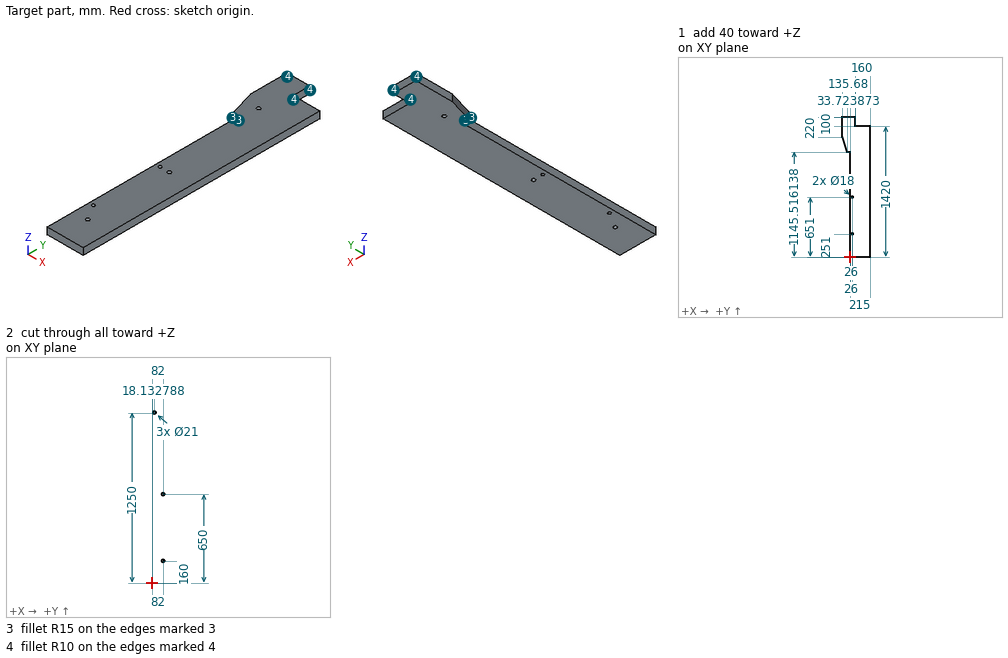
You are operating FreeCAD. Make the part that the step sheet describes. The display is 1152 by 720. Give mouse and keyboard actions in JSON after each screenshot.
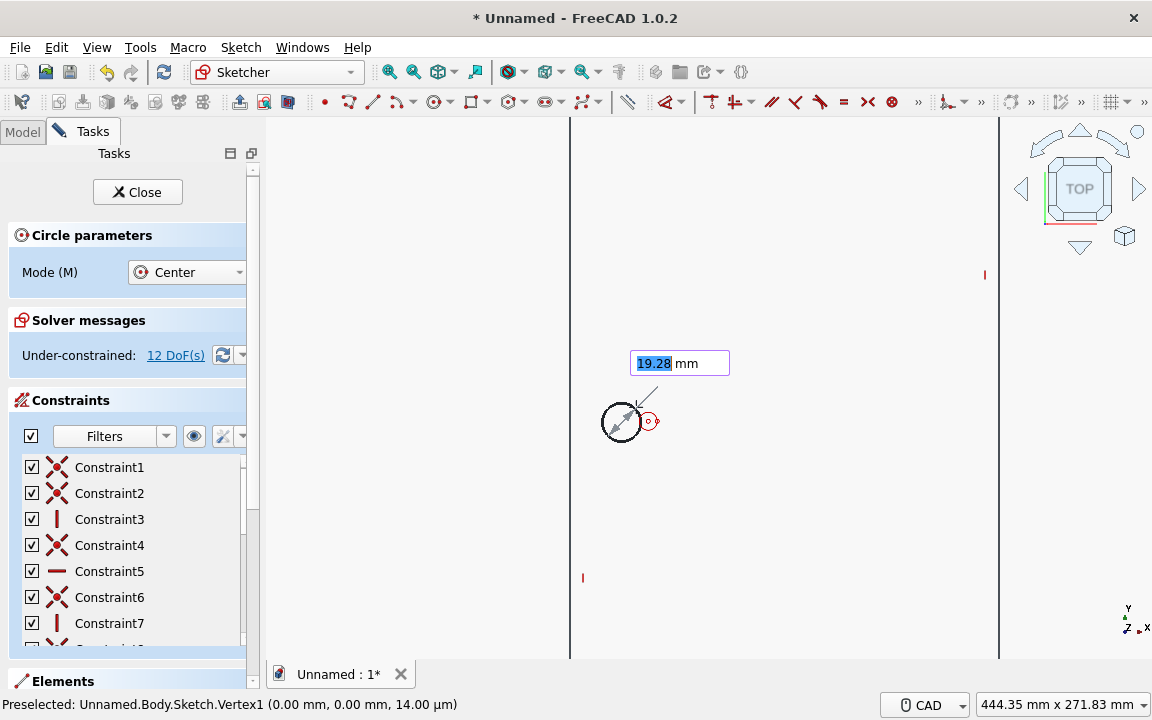
{"action": "left_click", "coordinate": [635, 406]}
{"action": "key", "text": "Escape"}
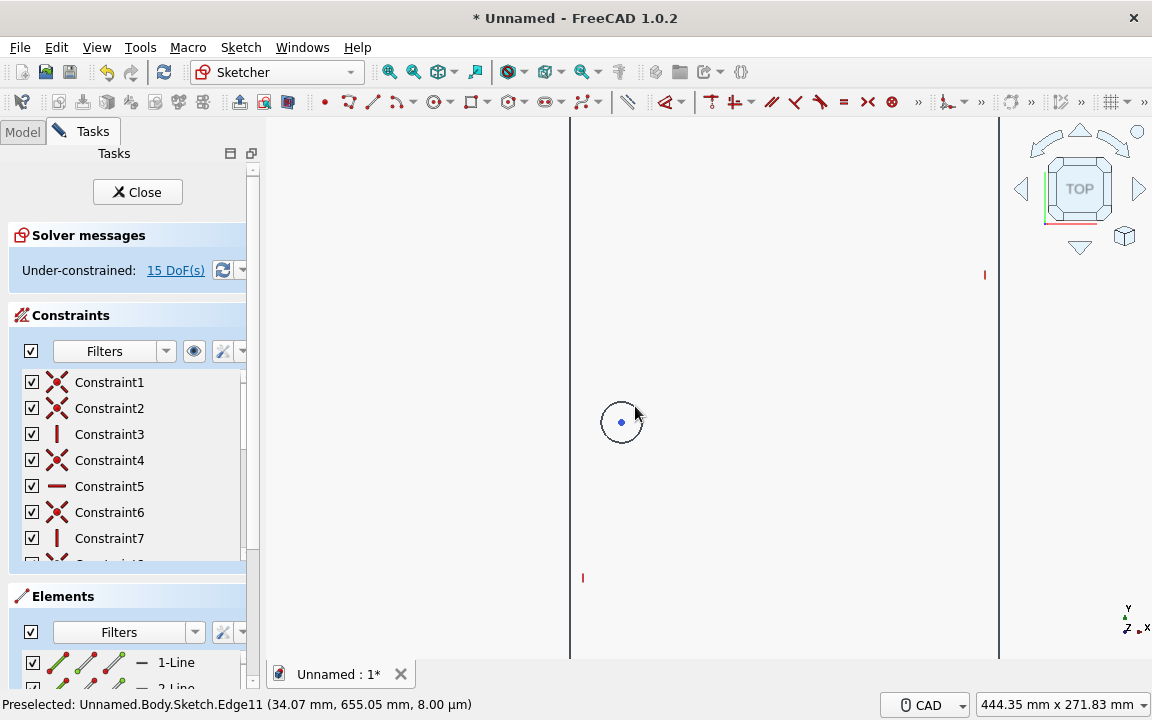
{"action": "scroll", "coordinate": [633, 411], "scroll_direction": "down", "scroll_amount": 11}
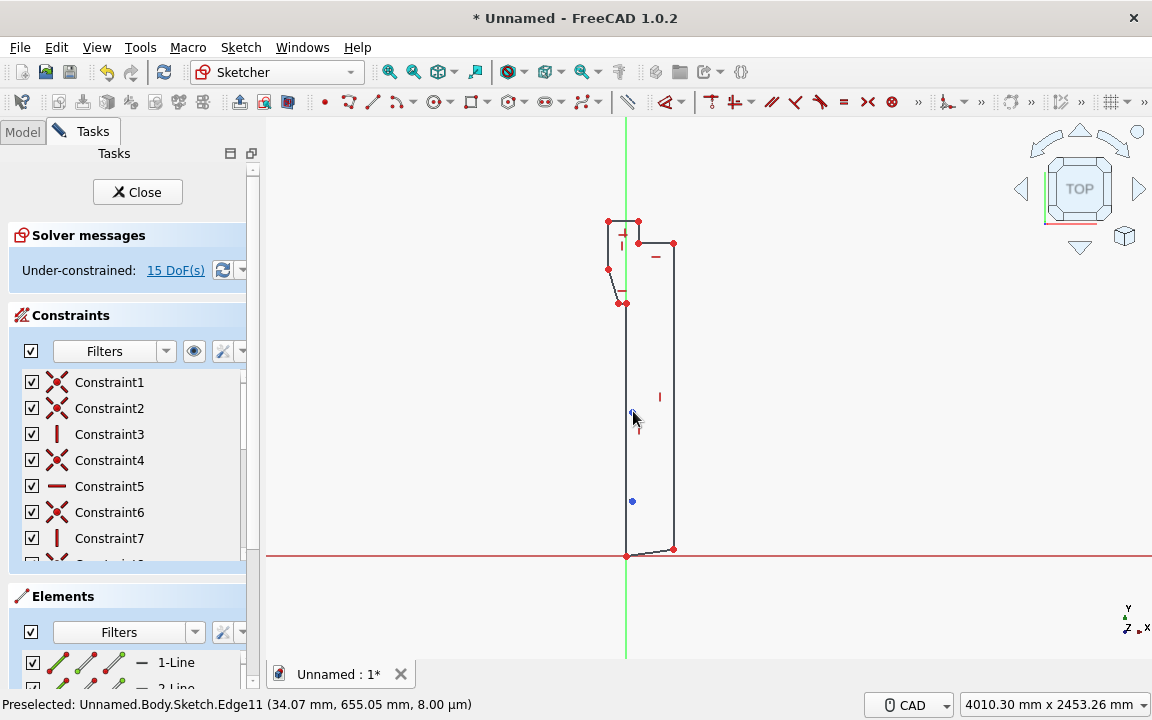
{"action": "scroll", "coordinate": [641, 554], "scroll_direction": "up", "scroll_amount": 10}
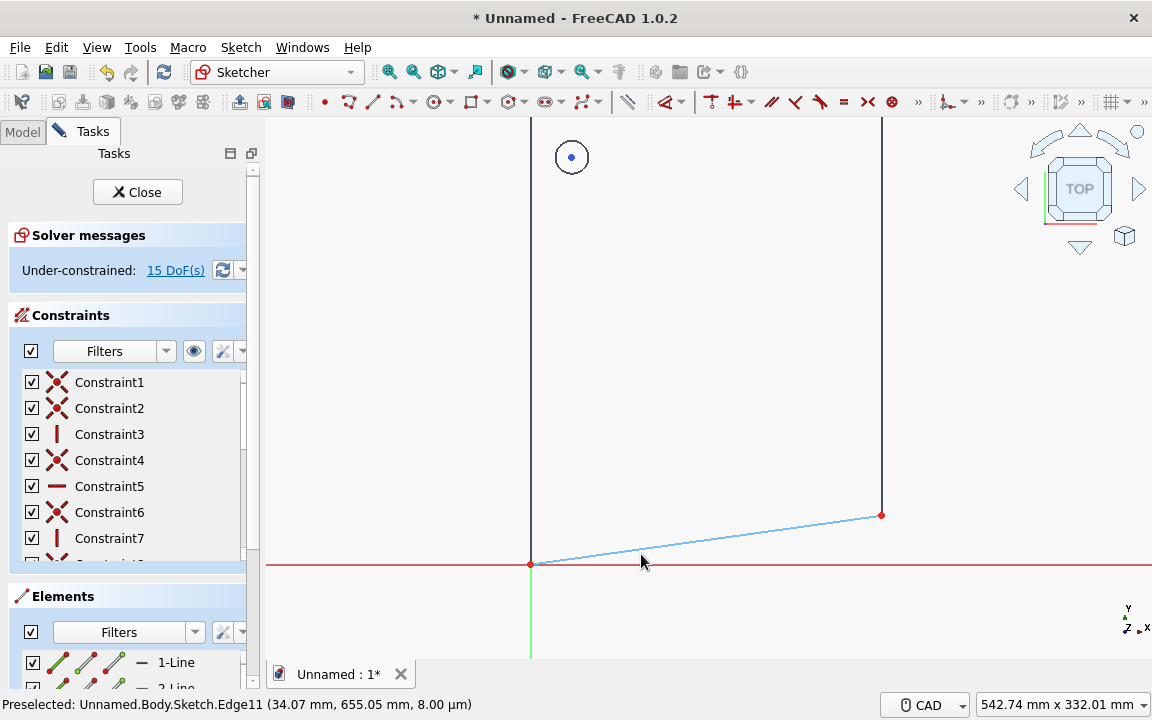
{"action": "left_click", "coordinate": [636, 550]}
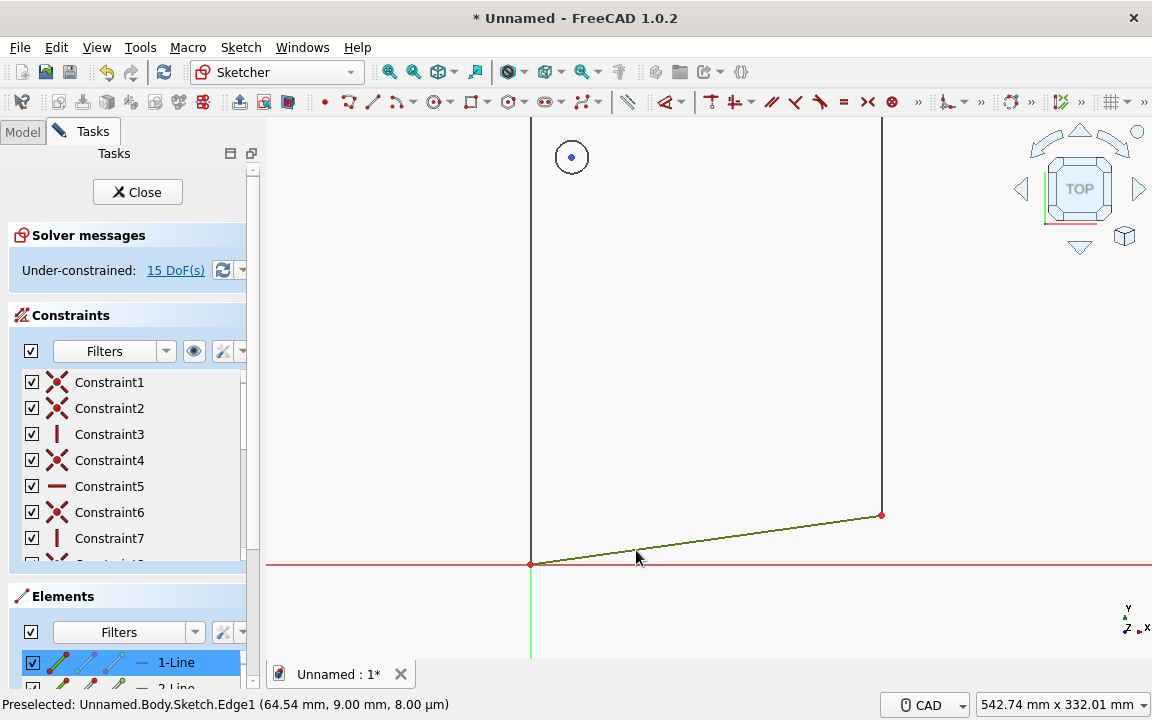
{"action": "key", "text": "h"}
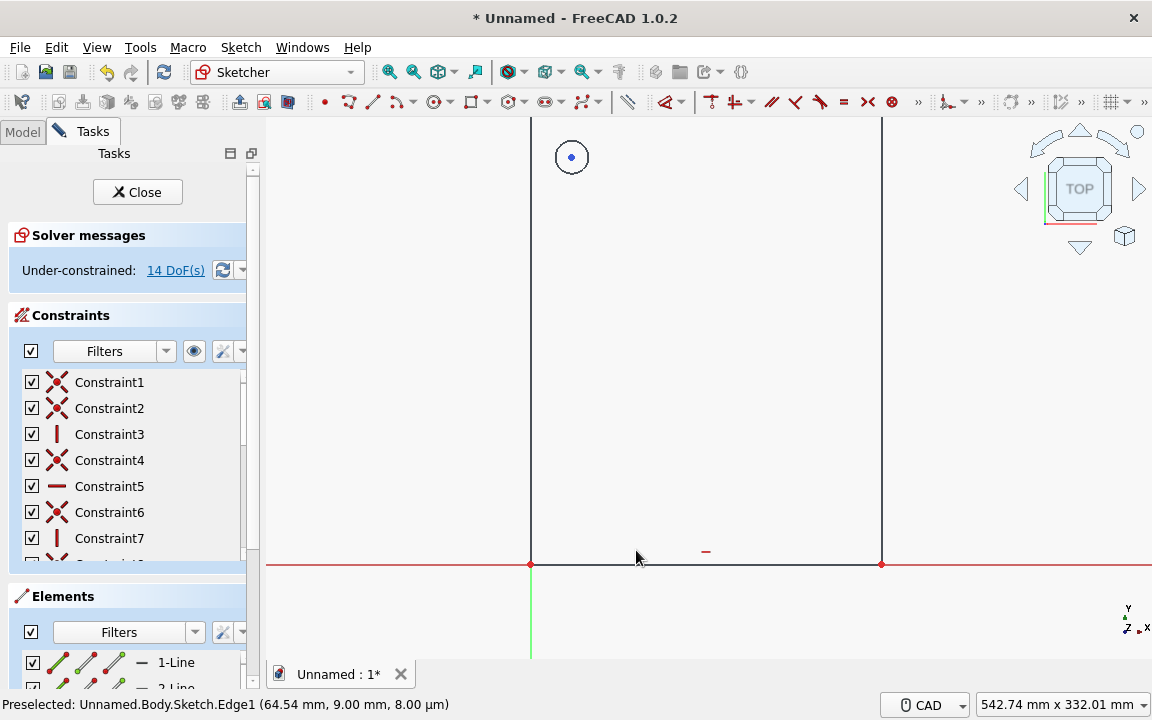
{"action": "left_click", "coordinate": [584, 146]}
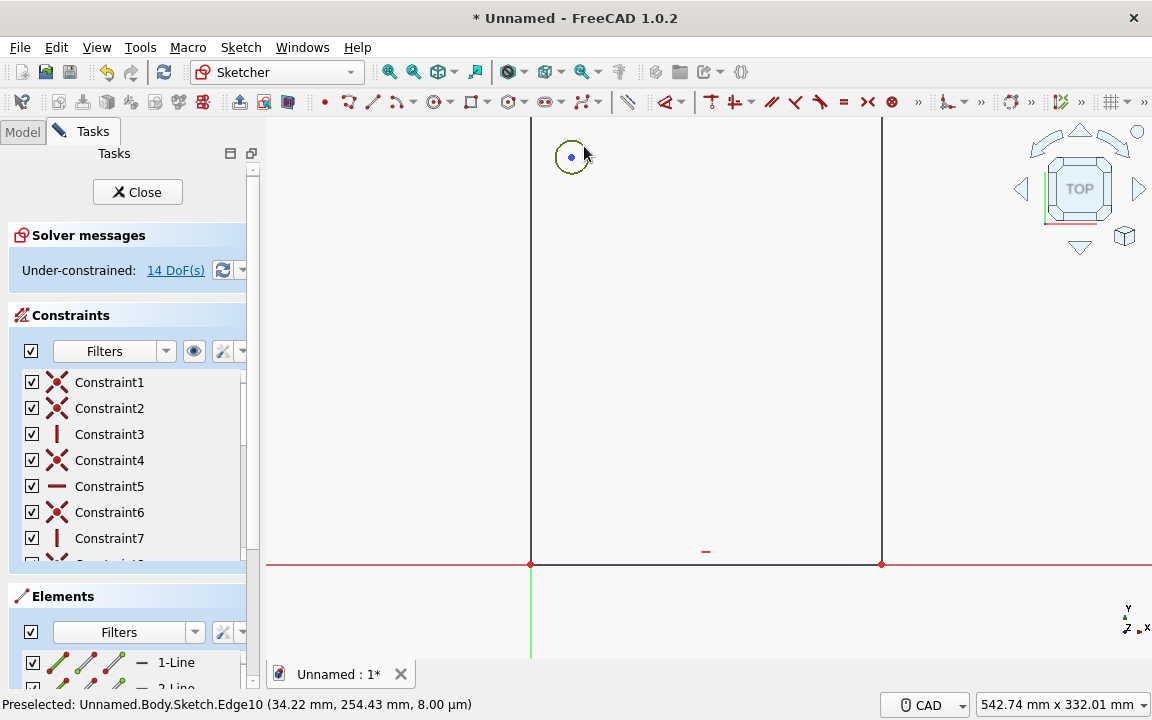
{"action": "scroll", "coordinate": [641, 555], "scroll_direction": "down", "scroll_amount": 10}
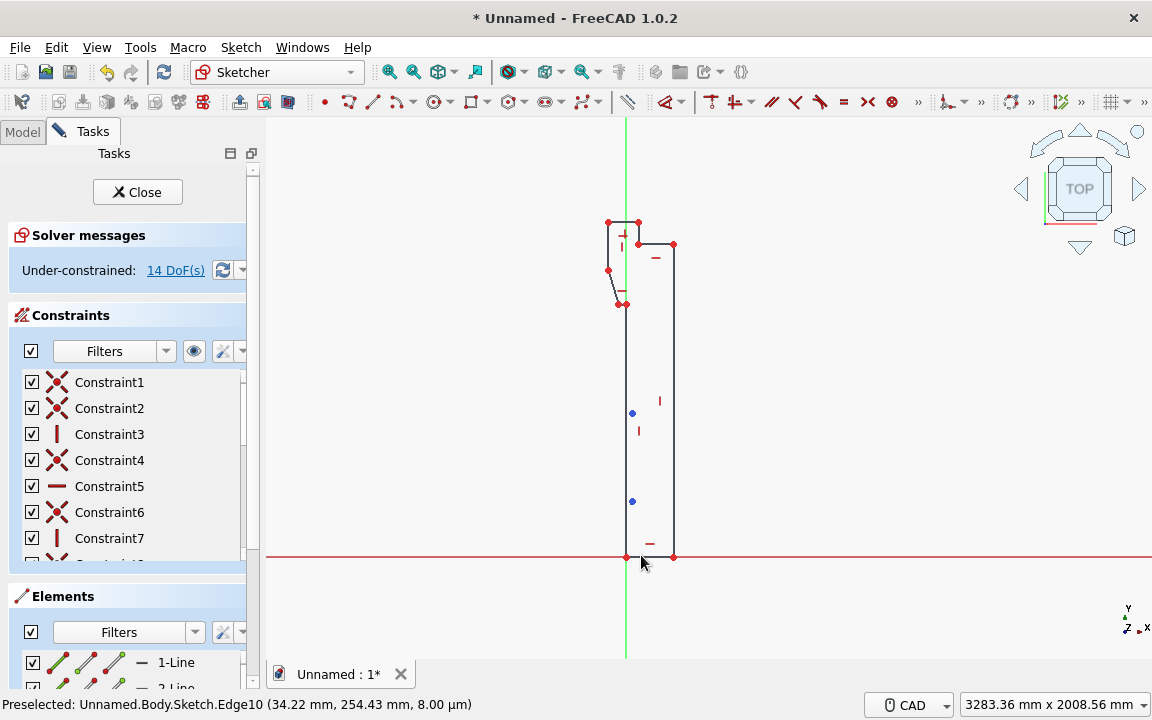
{"action": "scroll", "coordinate": [634, 412], "scroll_direction": "up", "scroll_amount": 10}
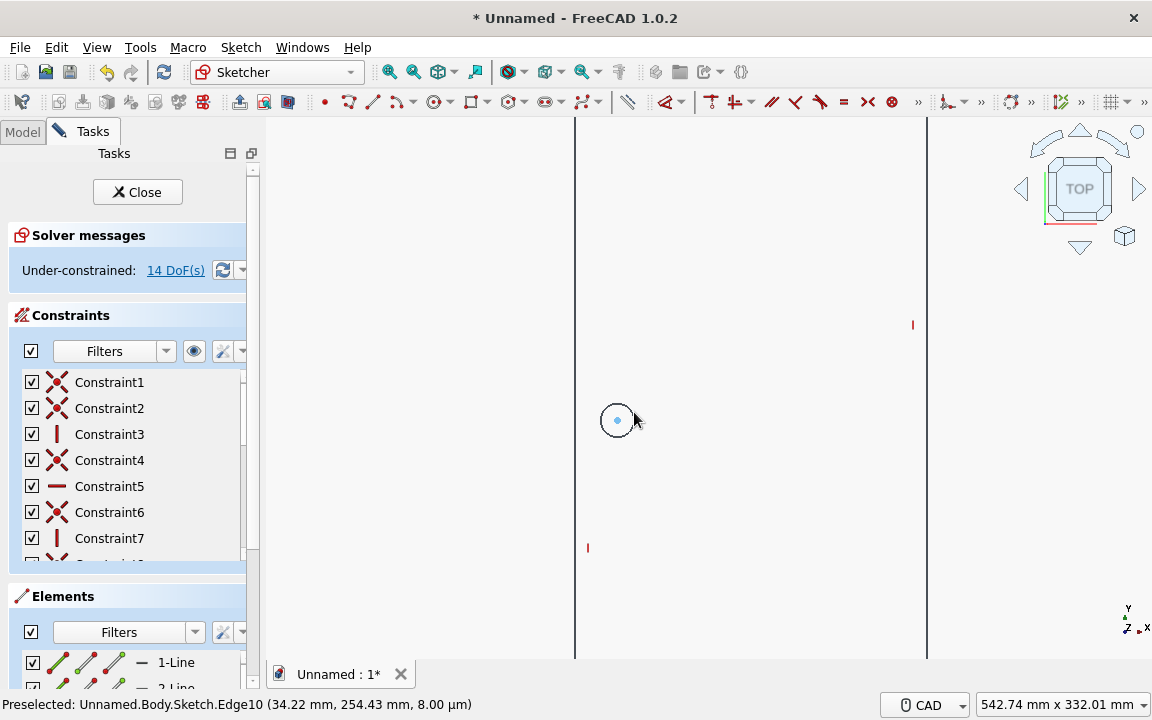
{"action": "left_click", "coordinate": [629, 409]}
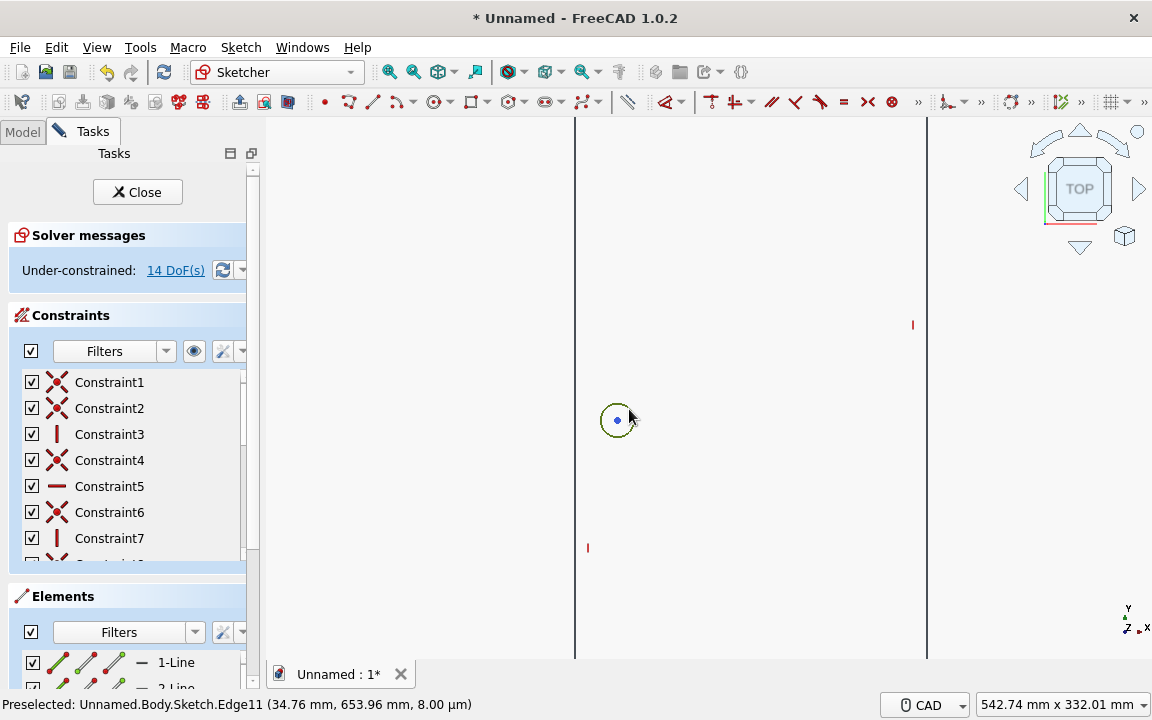
{"action": "key", "text": "e"}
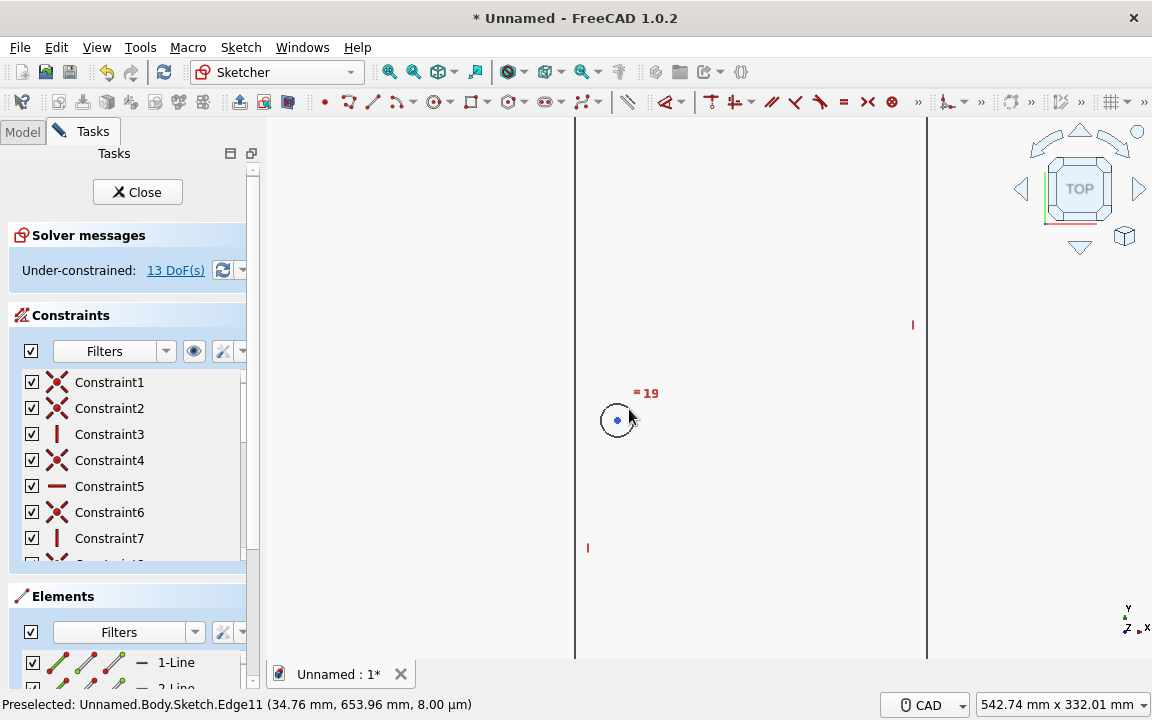
{"action": "key", "text": "d"}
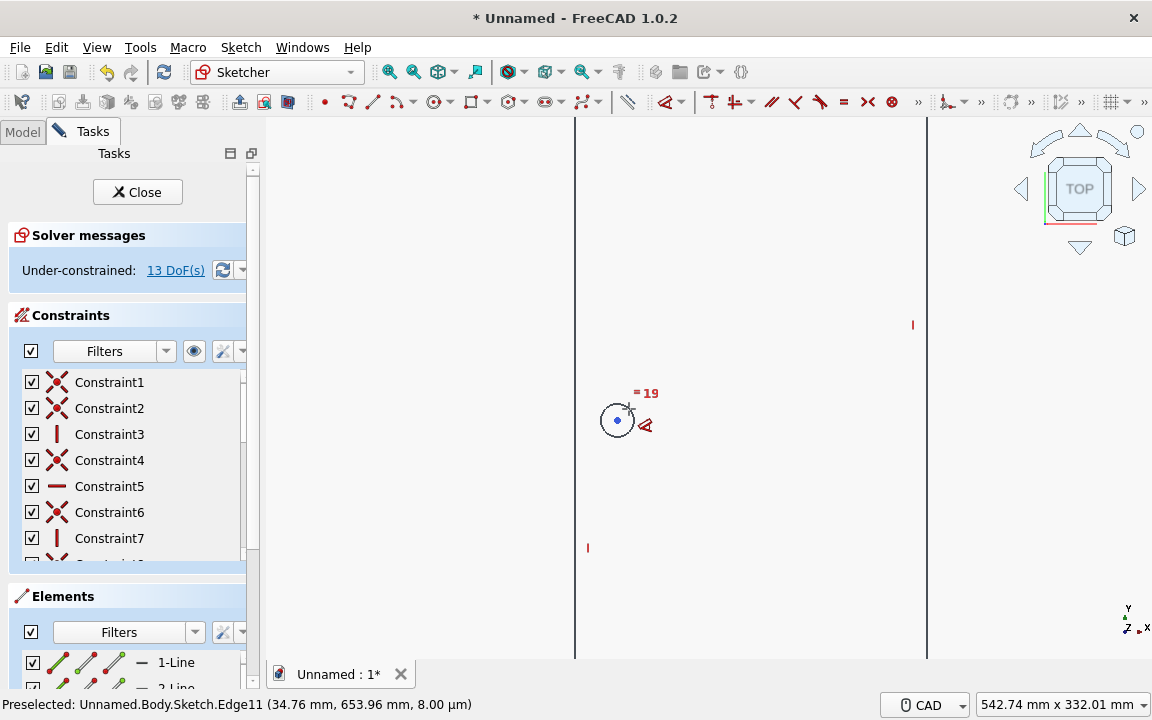
{"action": "scroll", "coordinate": [634, 411], "scroll_direction": "down", "scroll_amount": 10}